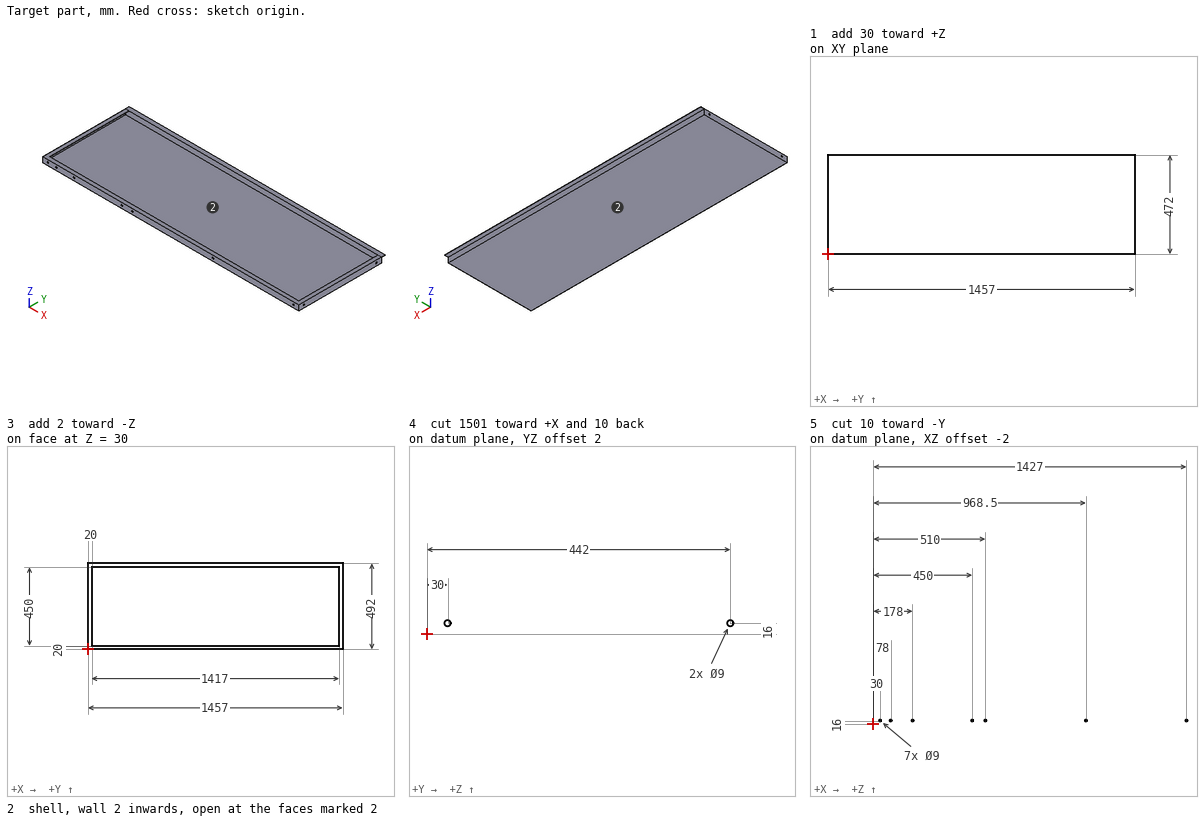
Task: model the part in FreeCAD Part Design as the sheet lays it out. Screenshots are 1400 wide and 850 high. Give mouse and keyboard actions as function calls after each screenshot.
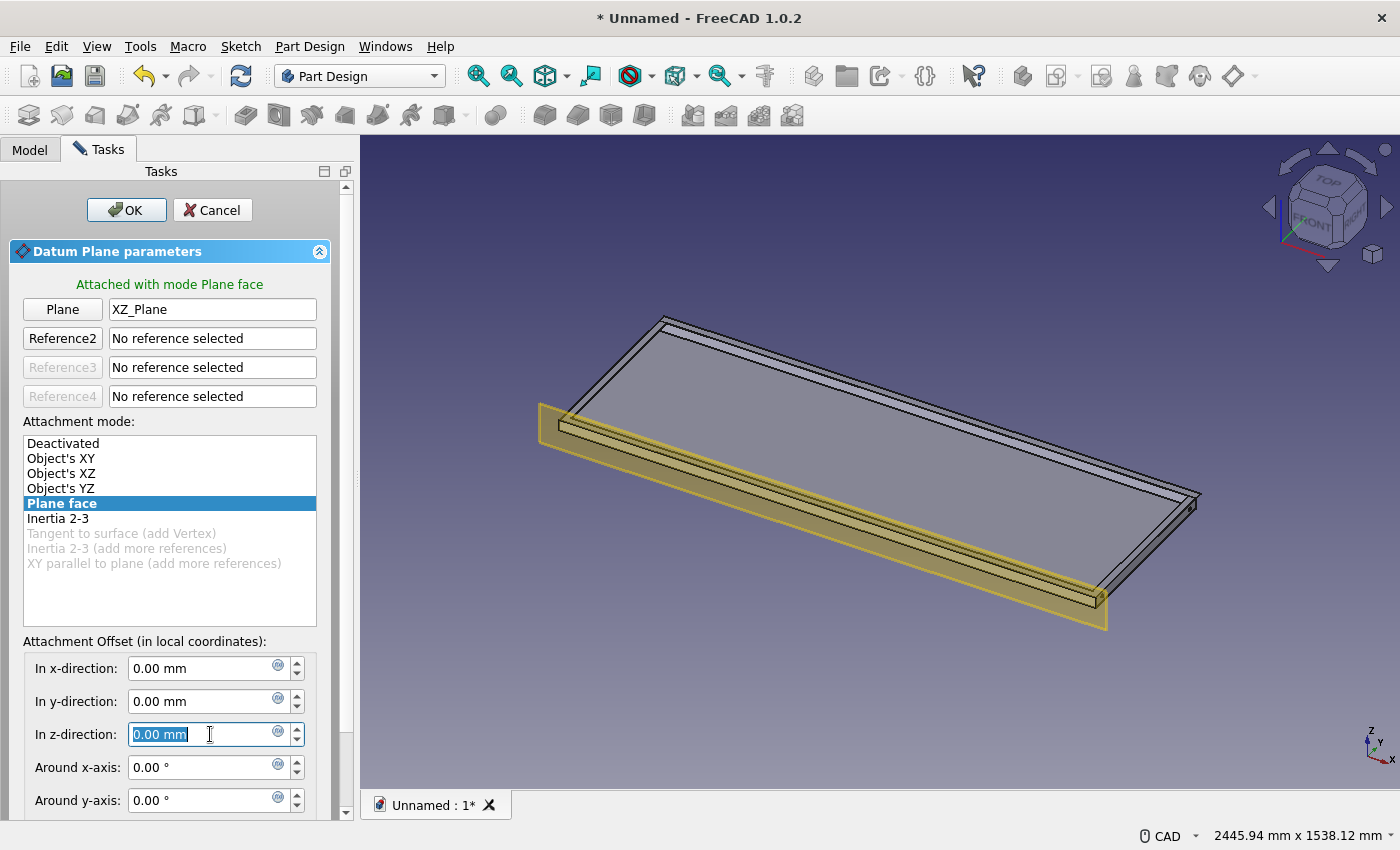
text(-2)
key(Tab)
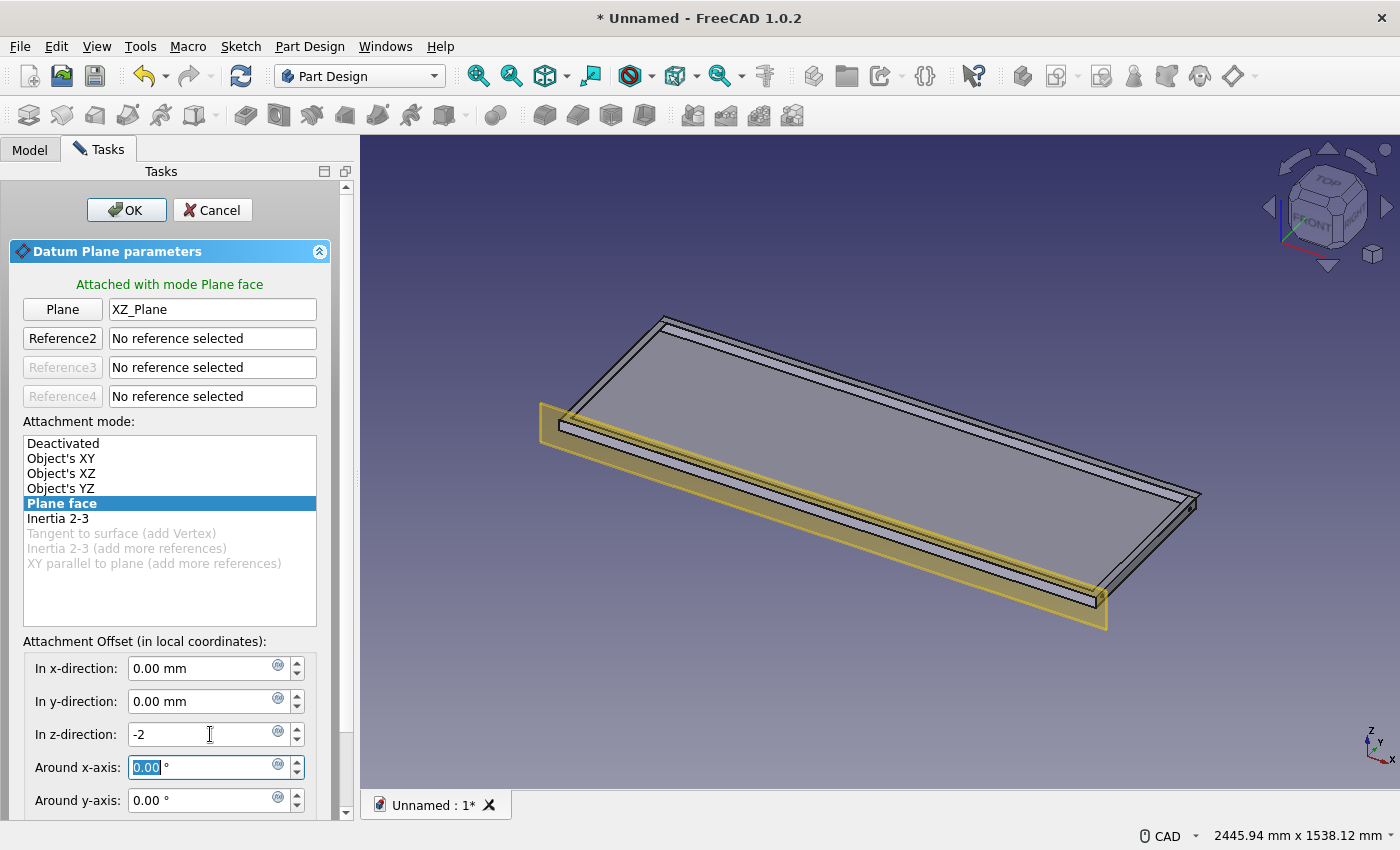
click(127, 210)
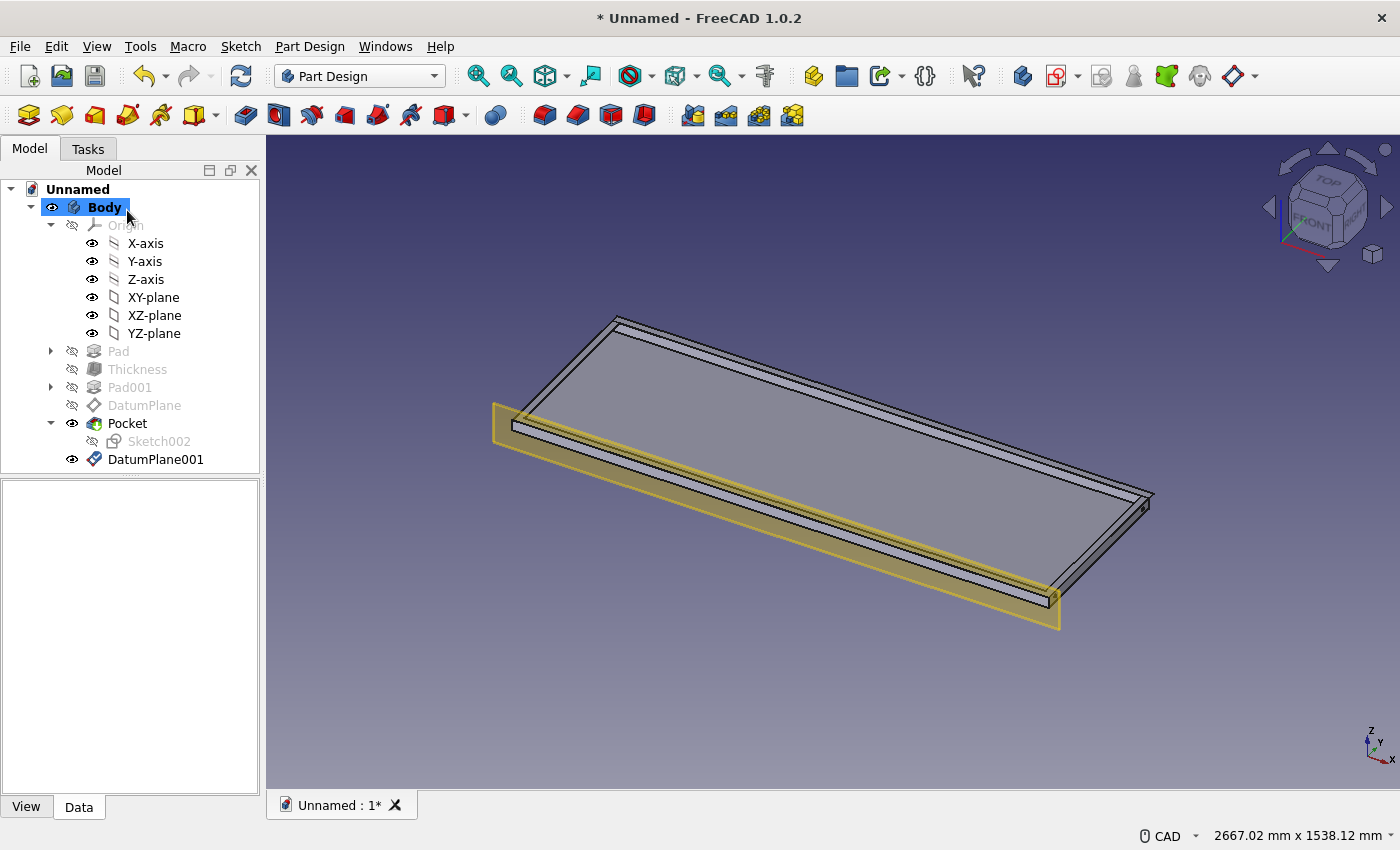
click(117, 459)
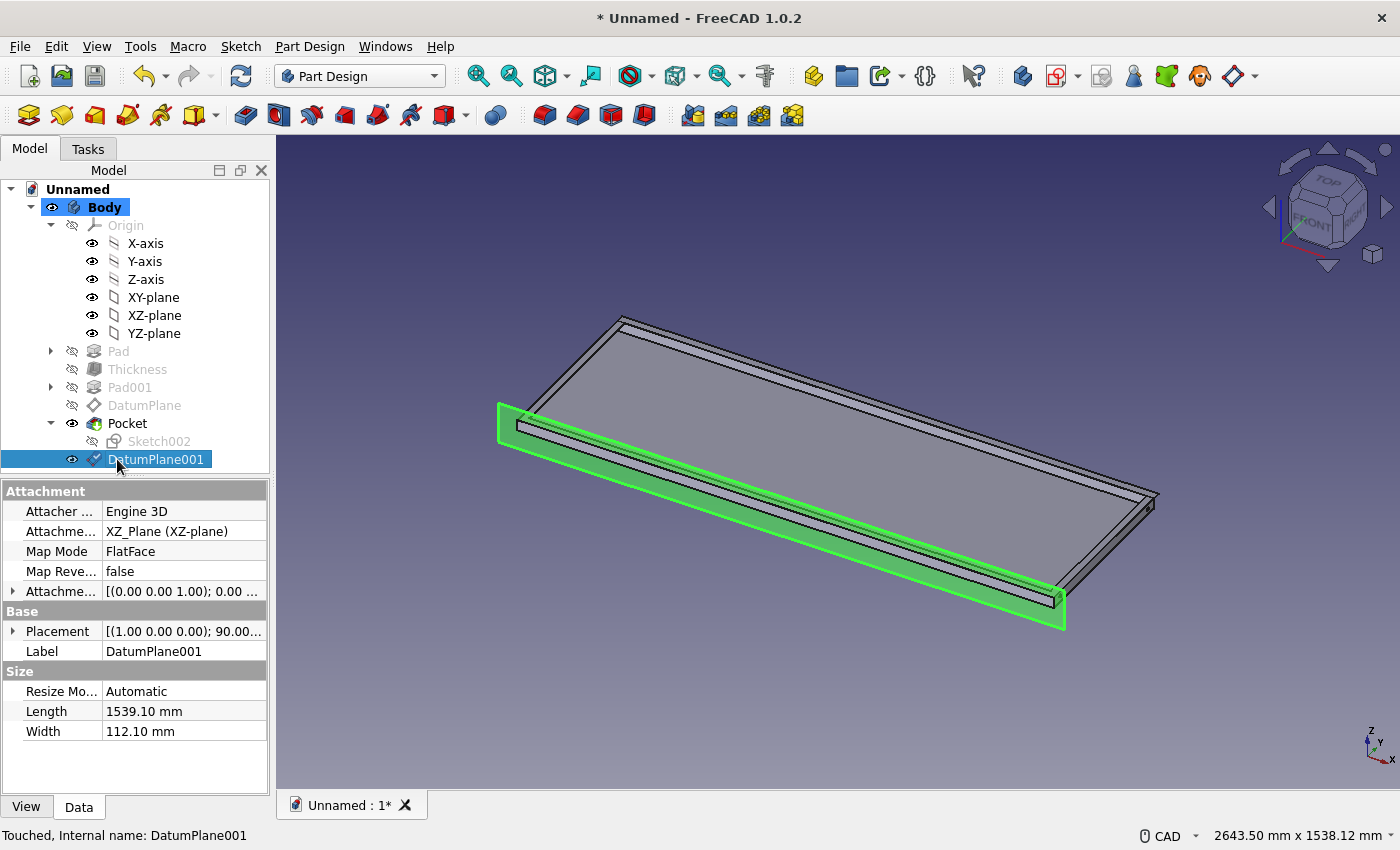
click(1056, 76)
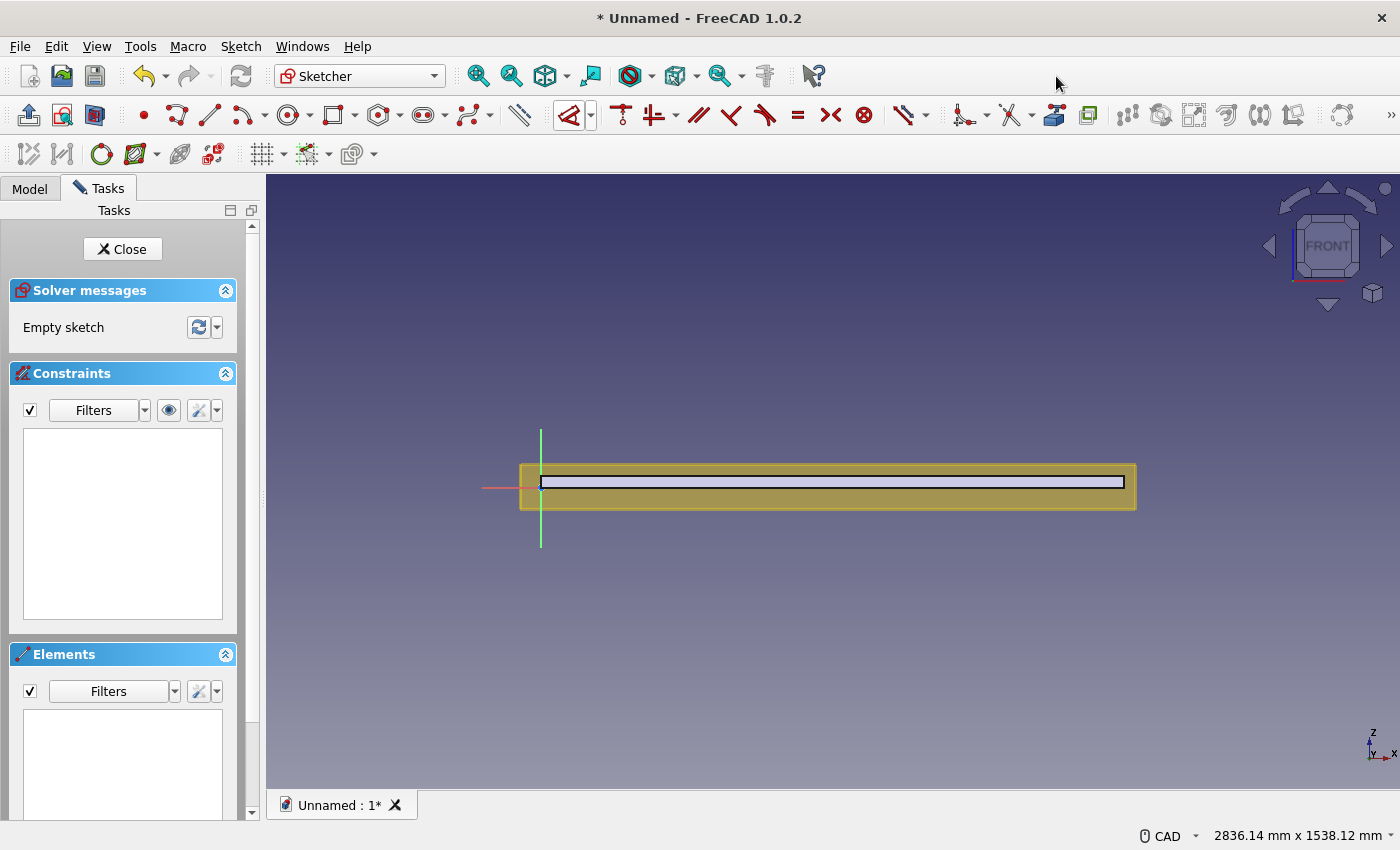
key(q)
key(s)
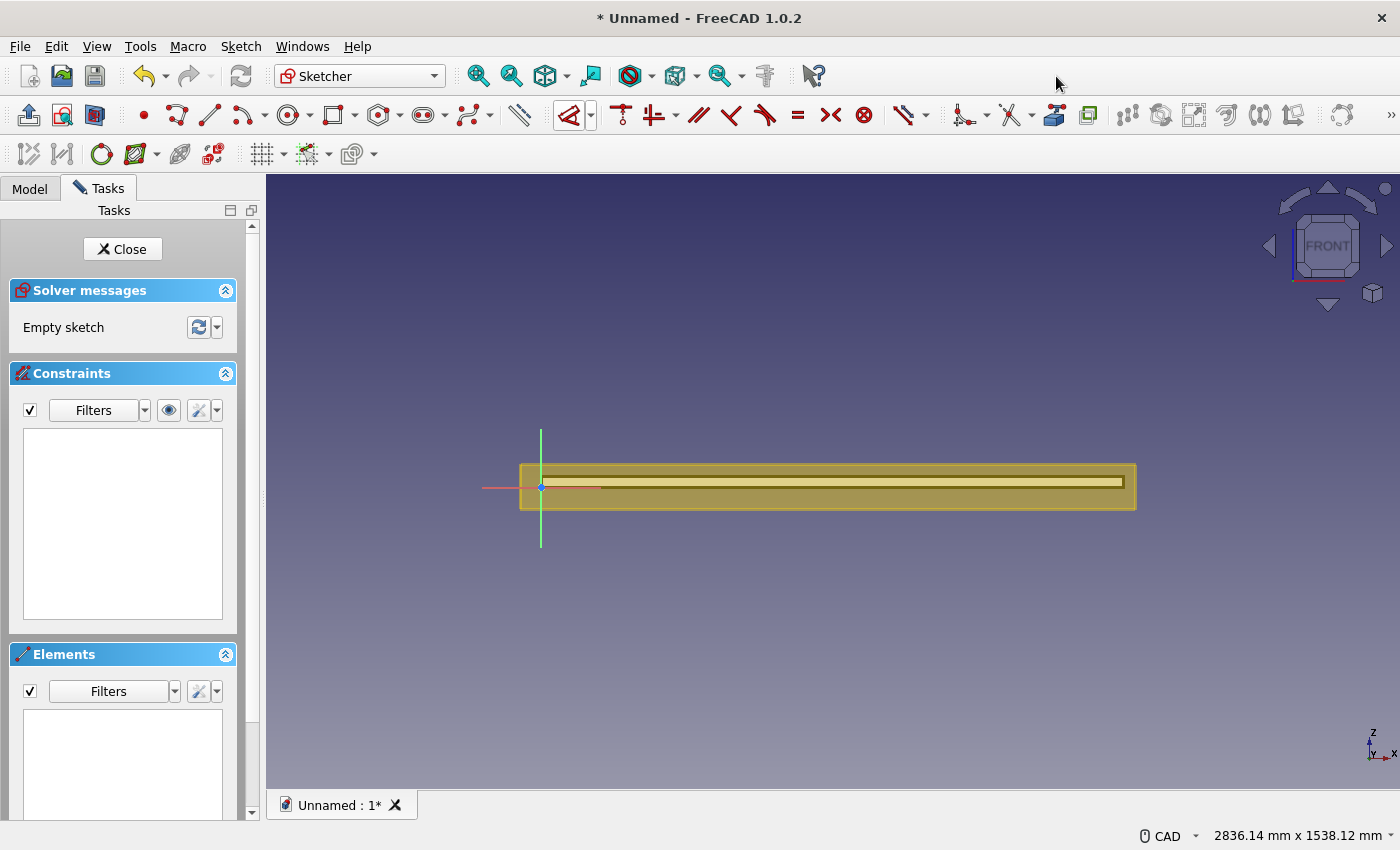
click(288, 116)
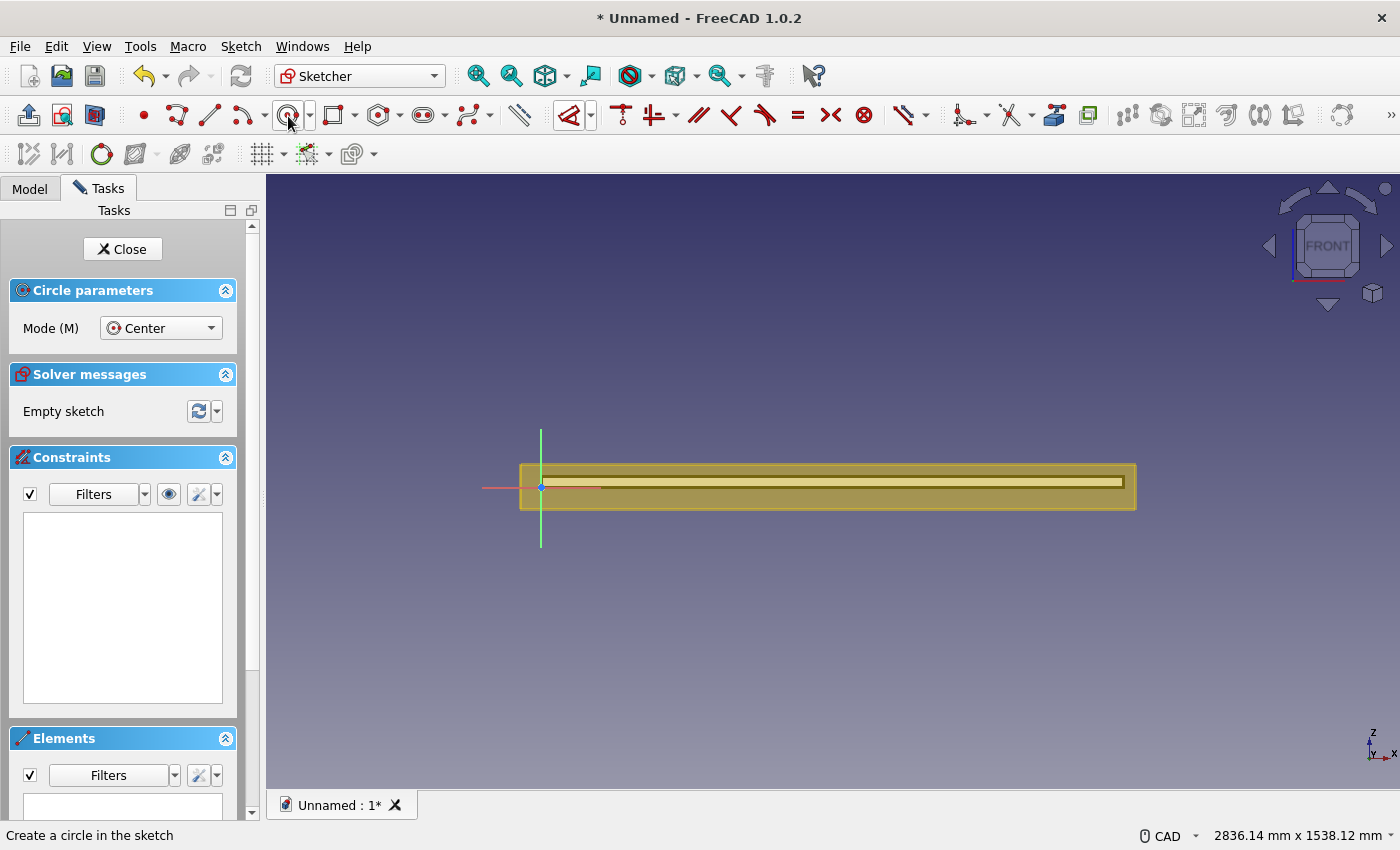
scroll(553, 482, up, 13)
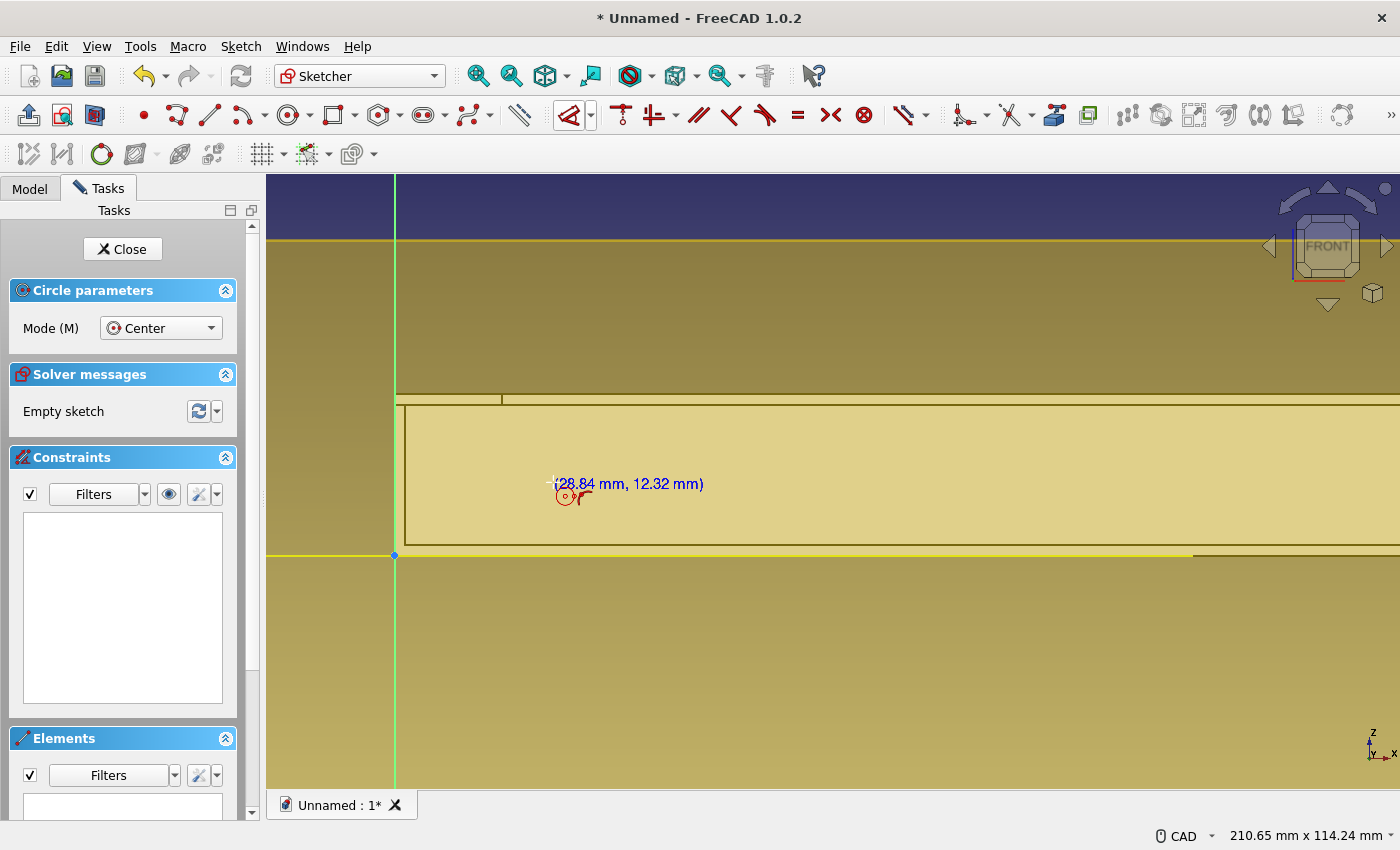
scroll(417, 480, down, 12)